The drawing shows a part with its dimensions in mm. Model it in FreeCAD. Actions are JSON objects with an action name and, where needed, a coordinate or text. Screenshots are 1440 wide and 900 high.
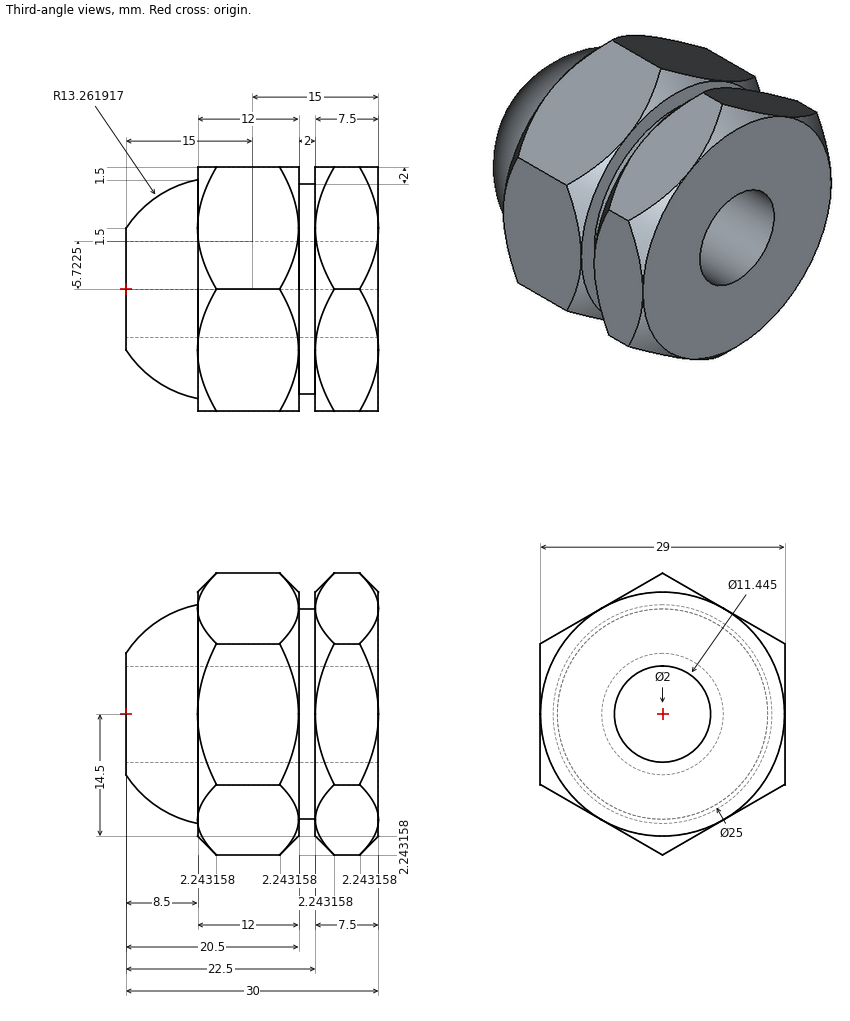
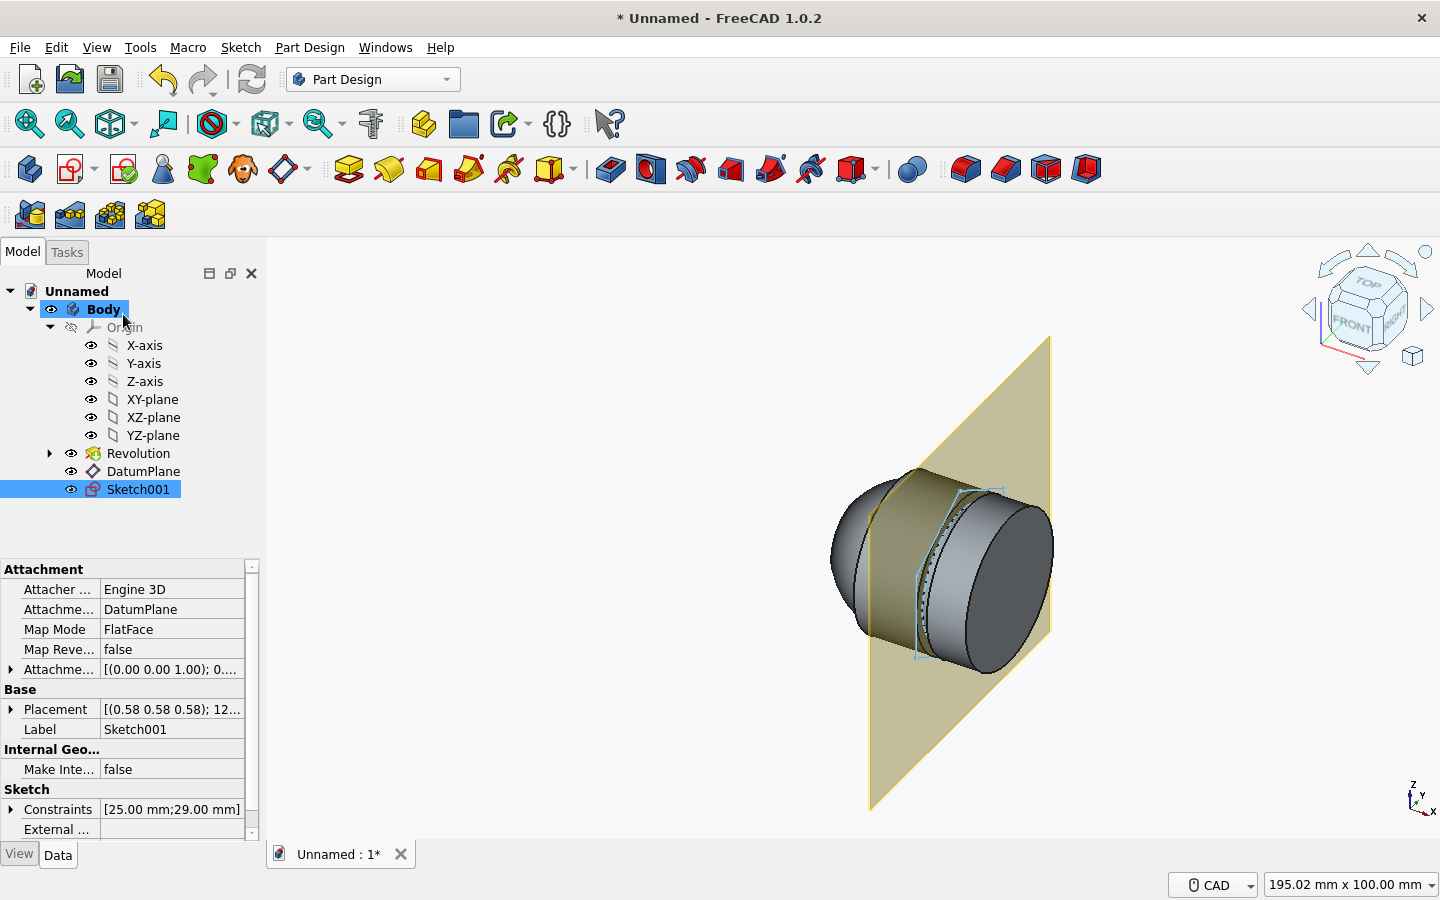
{"action": "left_click", "coordinate": [350, 170]}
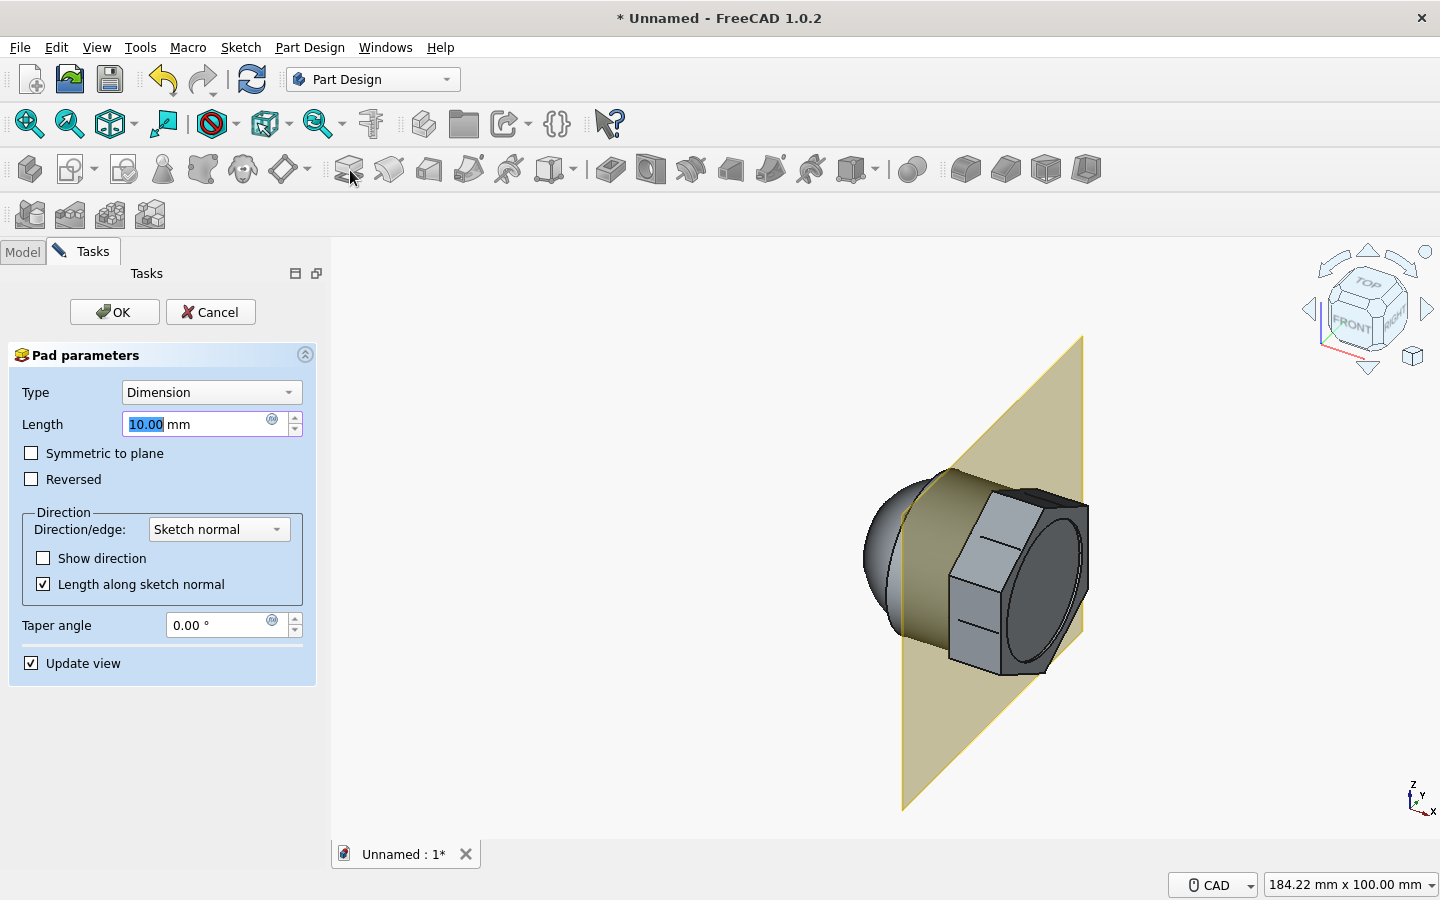
{"action": "type", "text": "12"}
{"action": "key", "text": "Tab"}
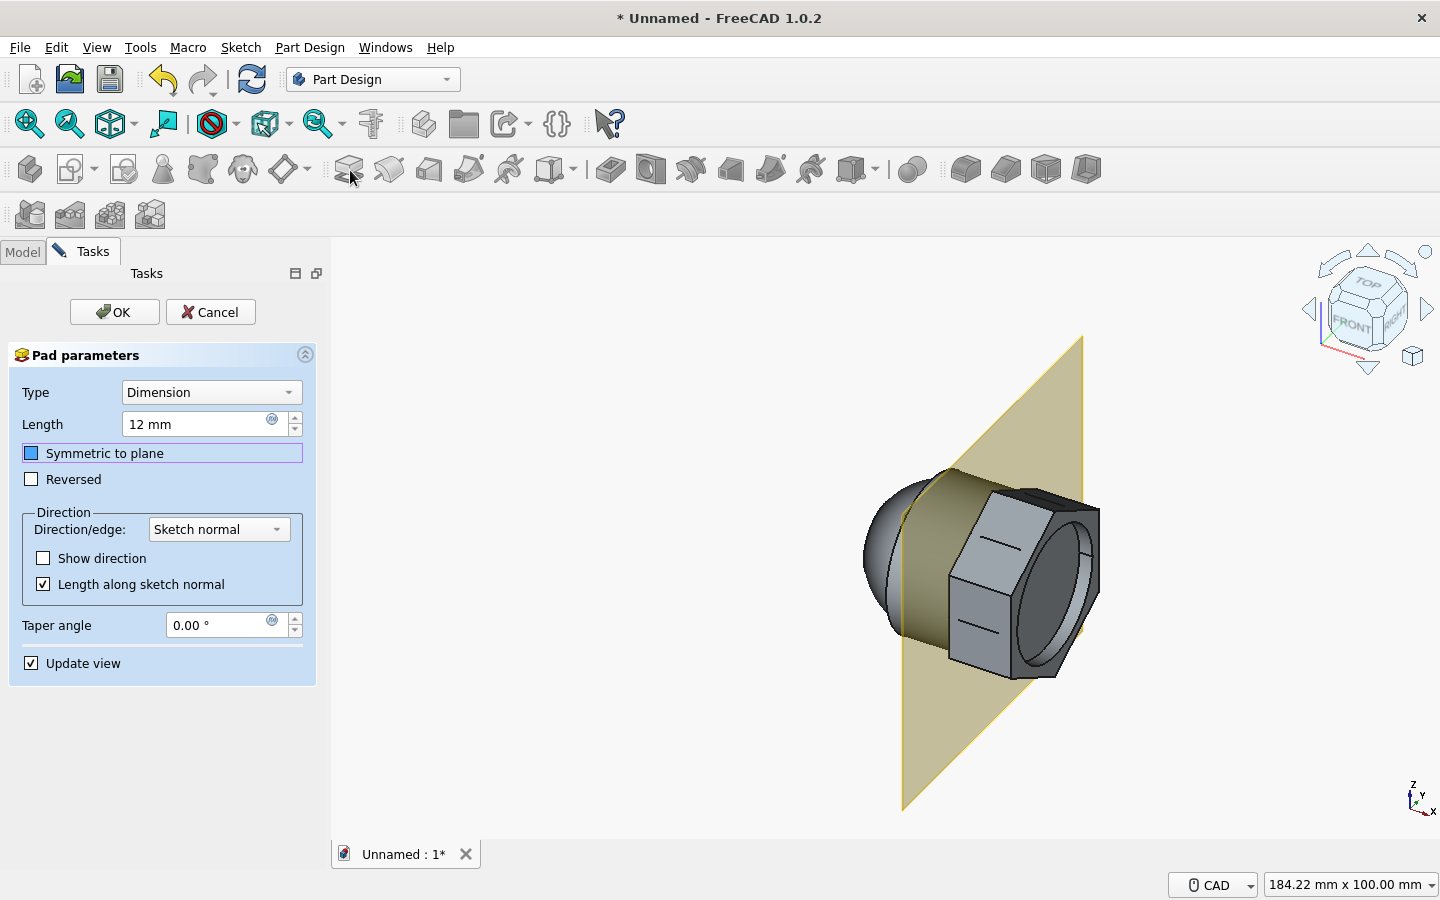
{"action": "left_click", "coordinate": [30, 479]}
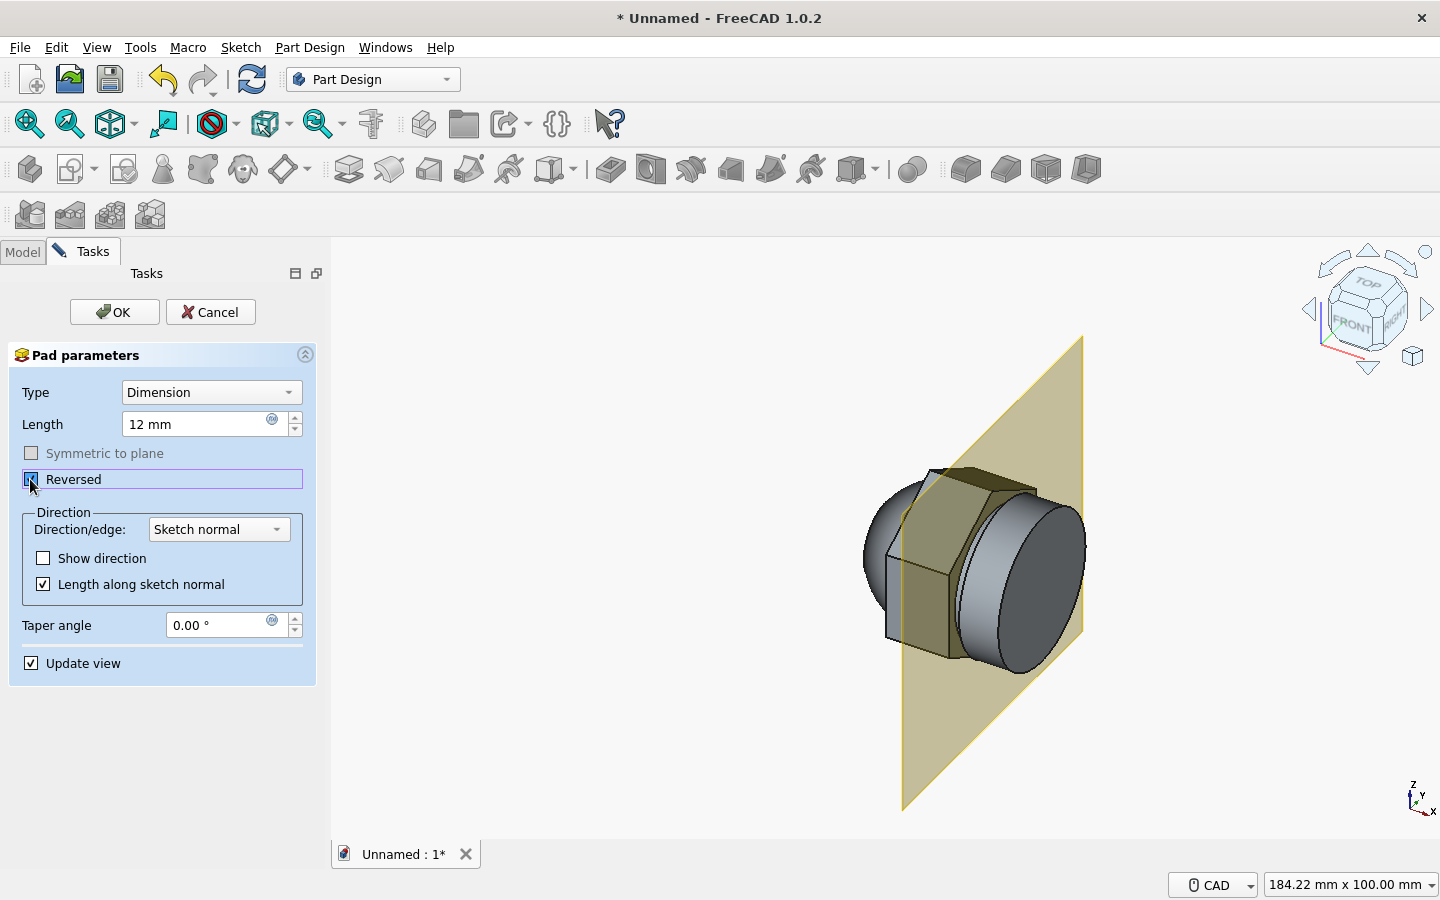
{"action": "left_click", "coordinate": [115, 312]}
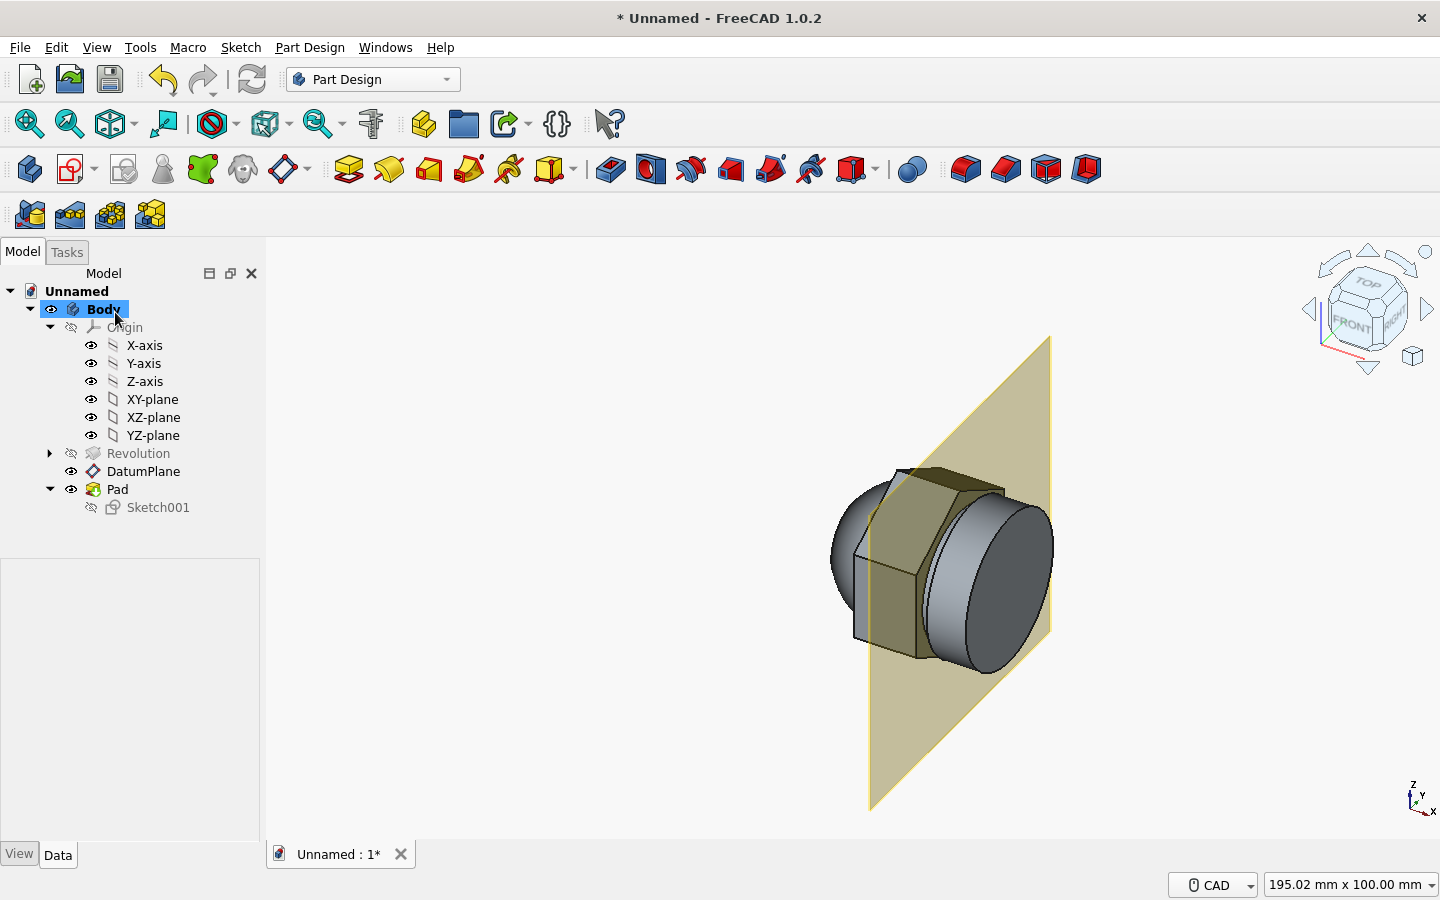
{"action": "left_click", "coordinate": [116, 471]}
{"action": "key", "text": "space"}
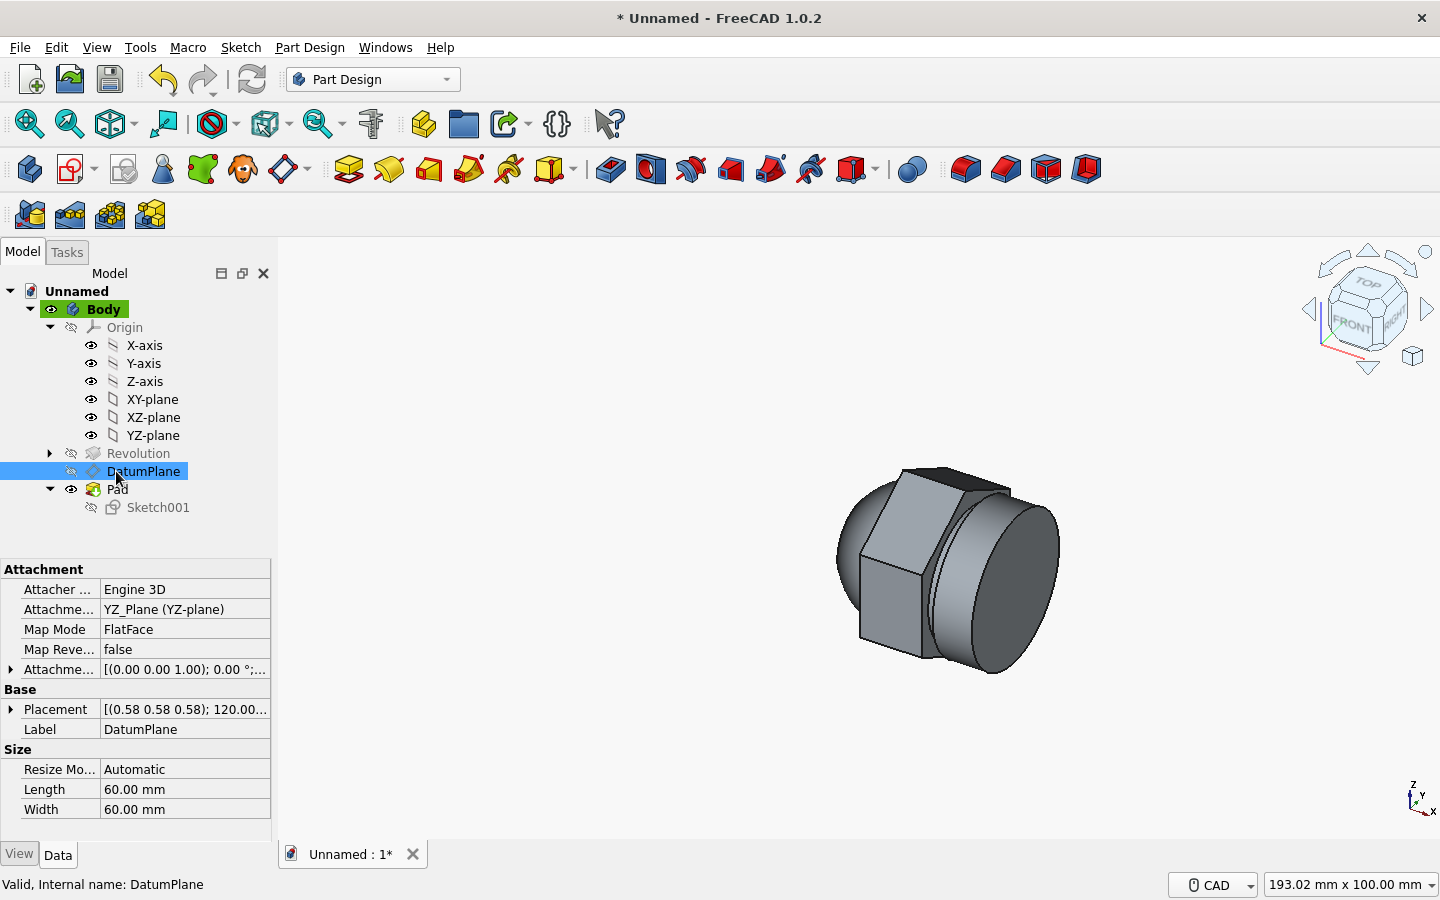
{"action": "left_click", "coordinate": [1015, 589]}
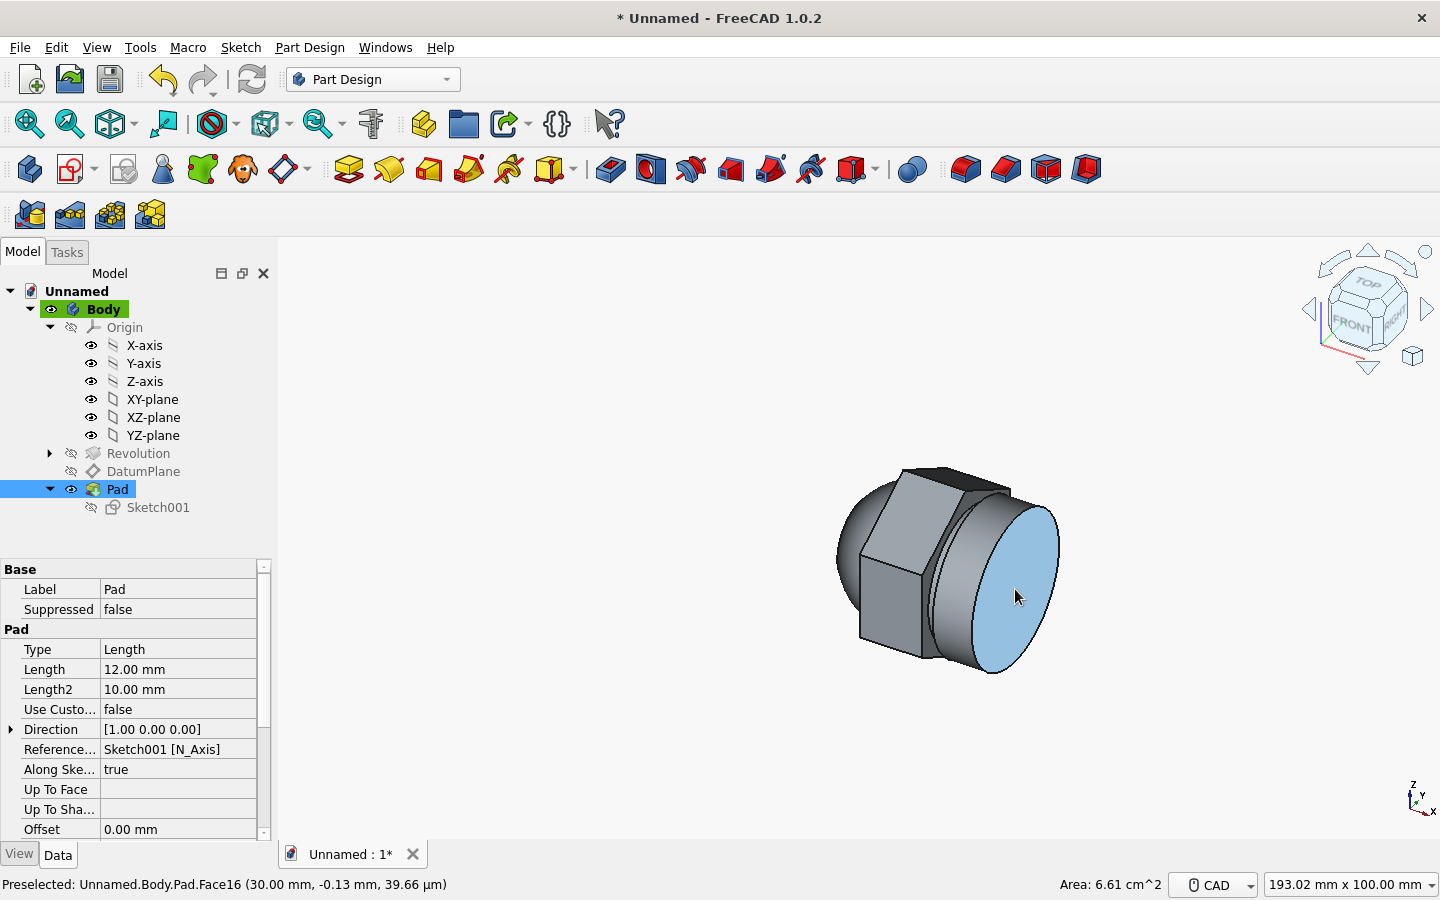
{"action": "left_click", "coordinate": [70, 170]}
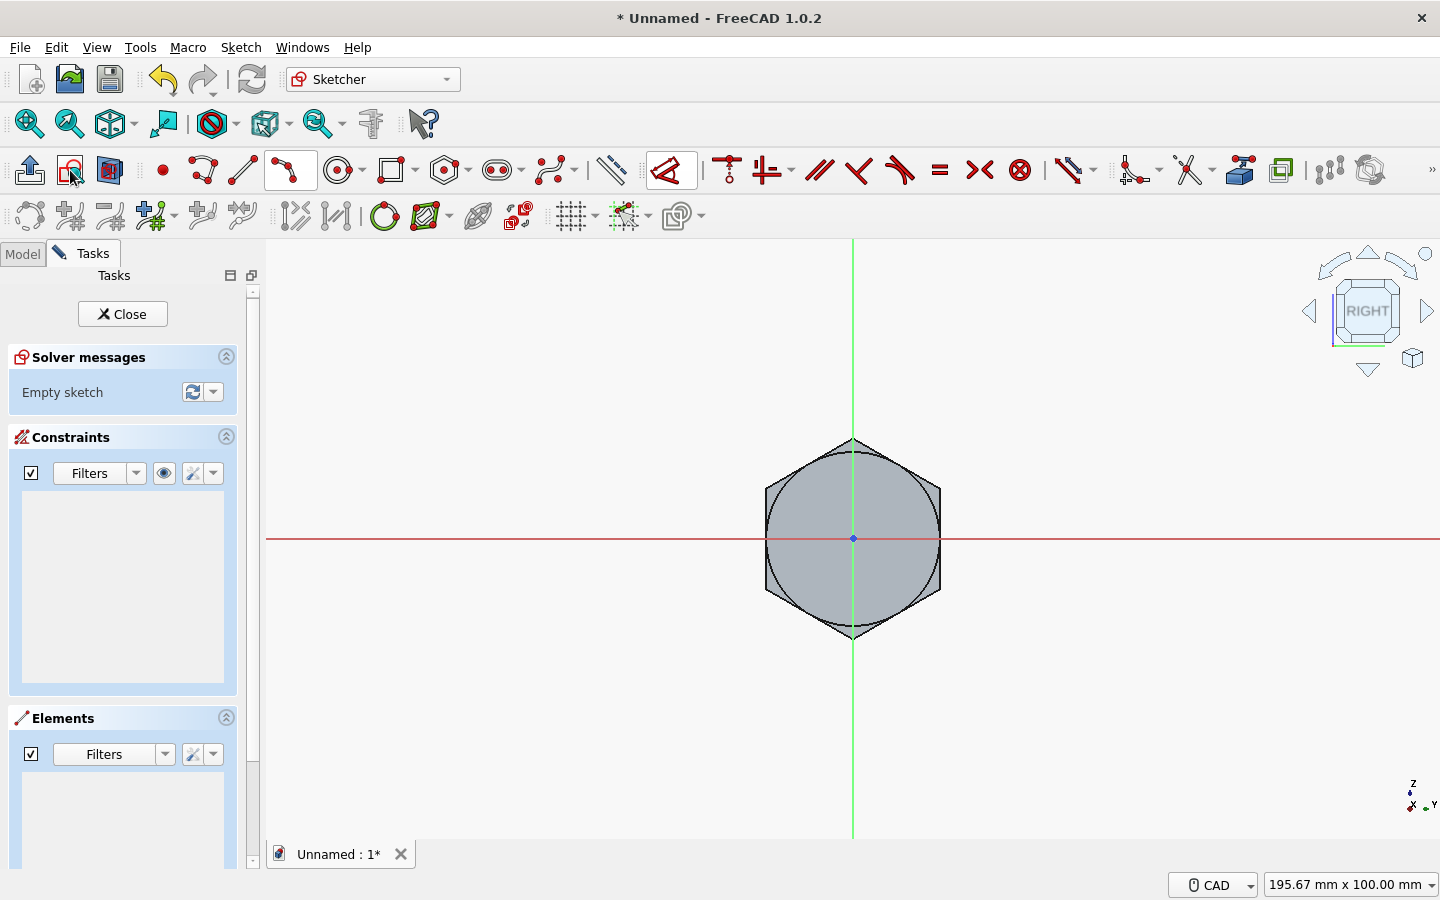
{"action": "scroll", "coordinate": [936, 539], "scroll_direction": "up", "scroll_amount": 3}